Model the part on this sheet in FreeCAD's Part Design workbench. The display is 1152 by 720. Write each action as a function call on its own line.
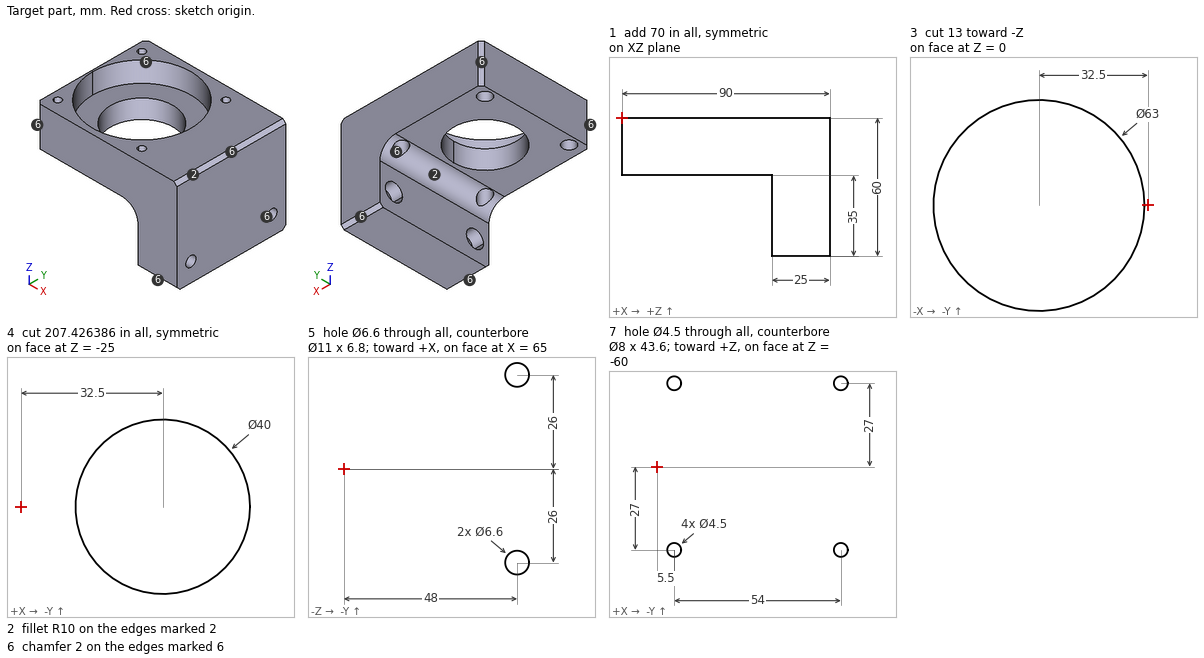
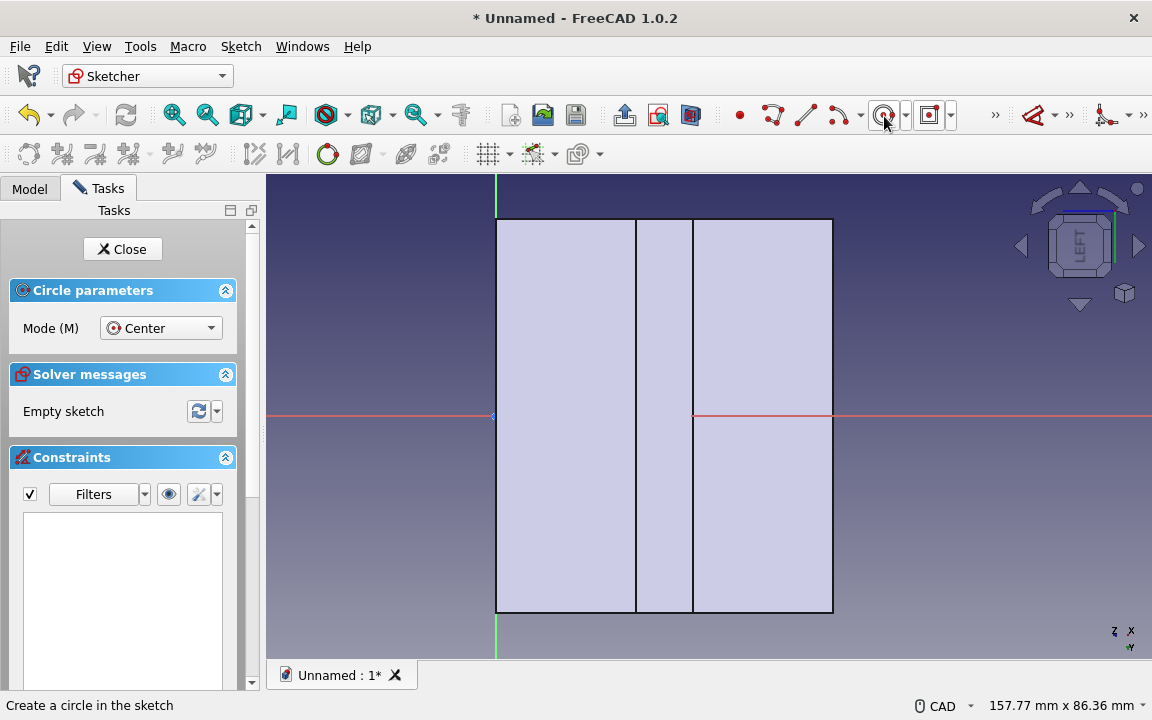
scroll(766, 562, up, 2)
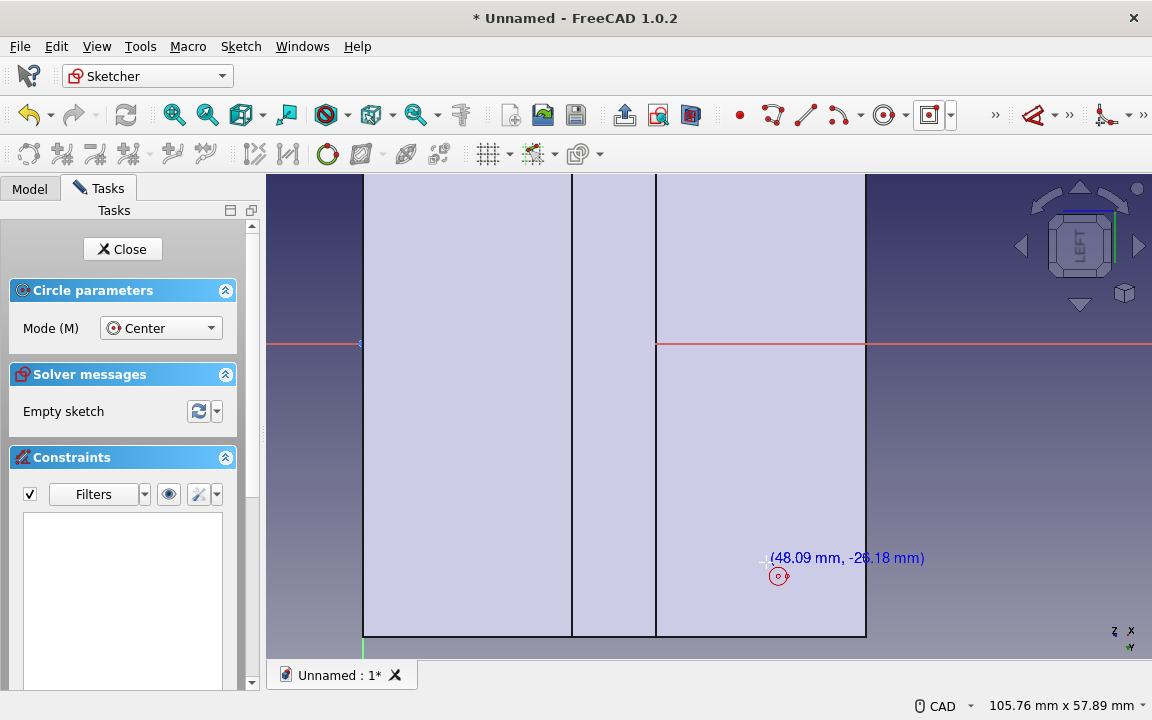
click(765, 562)
move(785, 542)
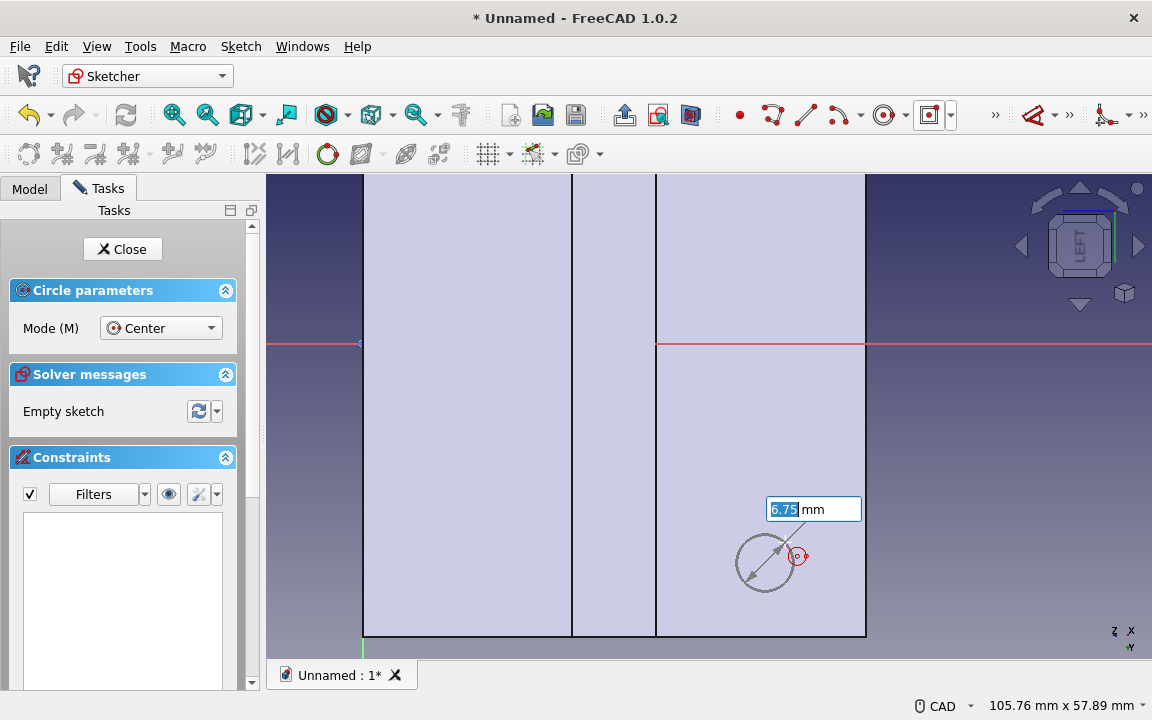
text(6.6)
key(Return)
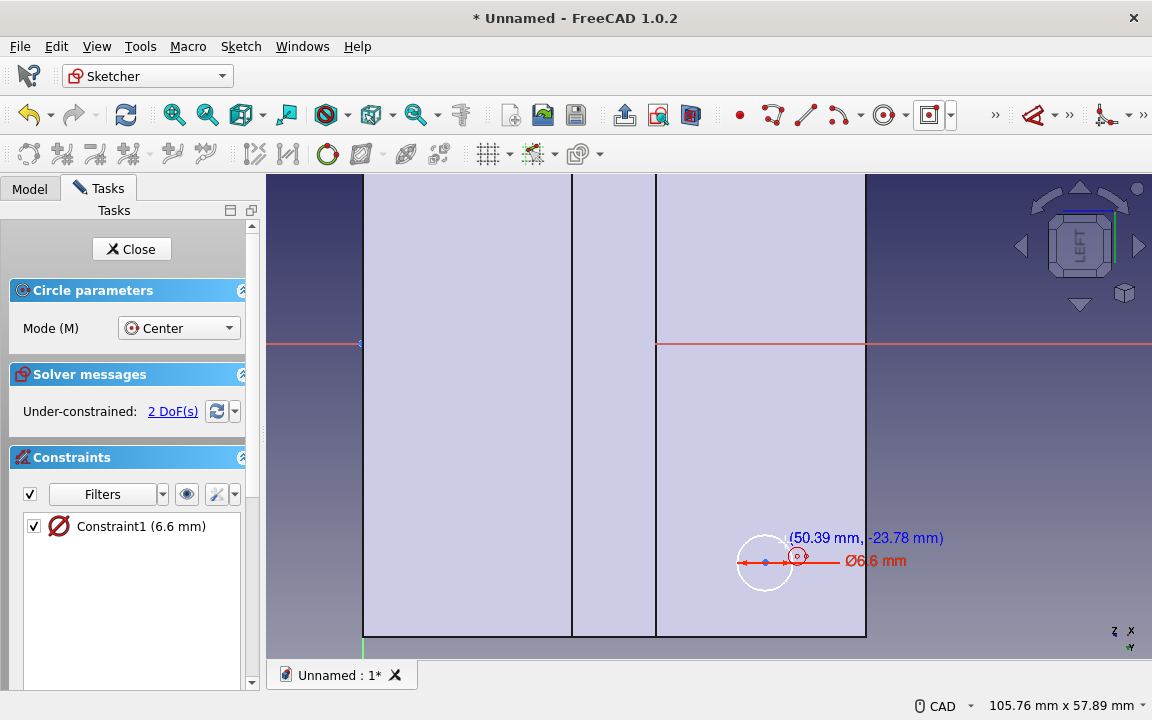
scroll(768, 564, down, 2)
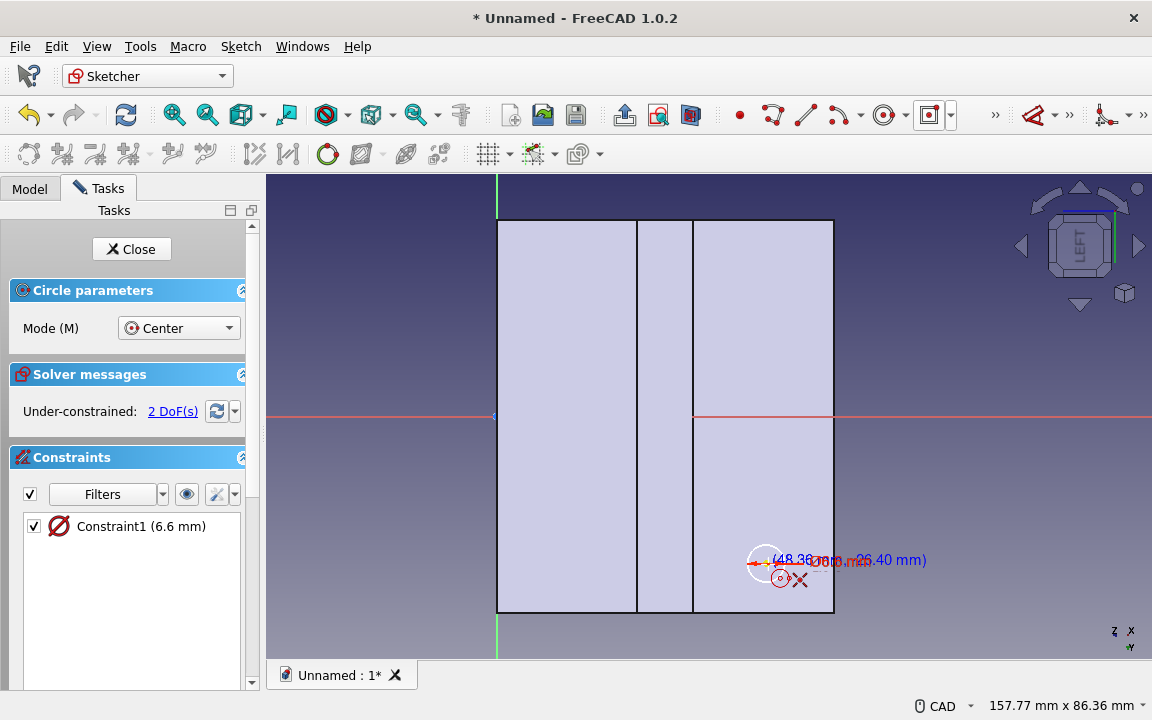
scroll(766, 271, up, 2)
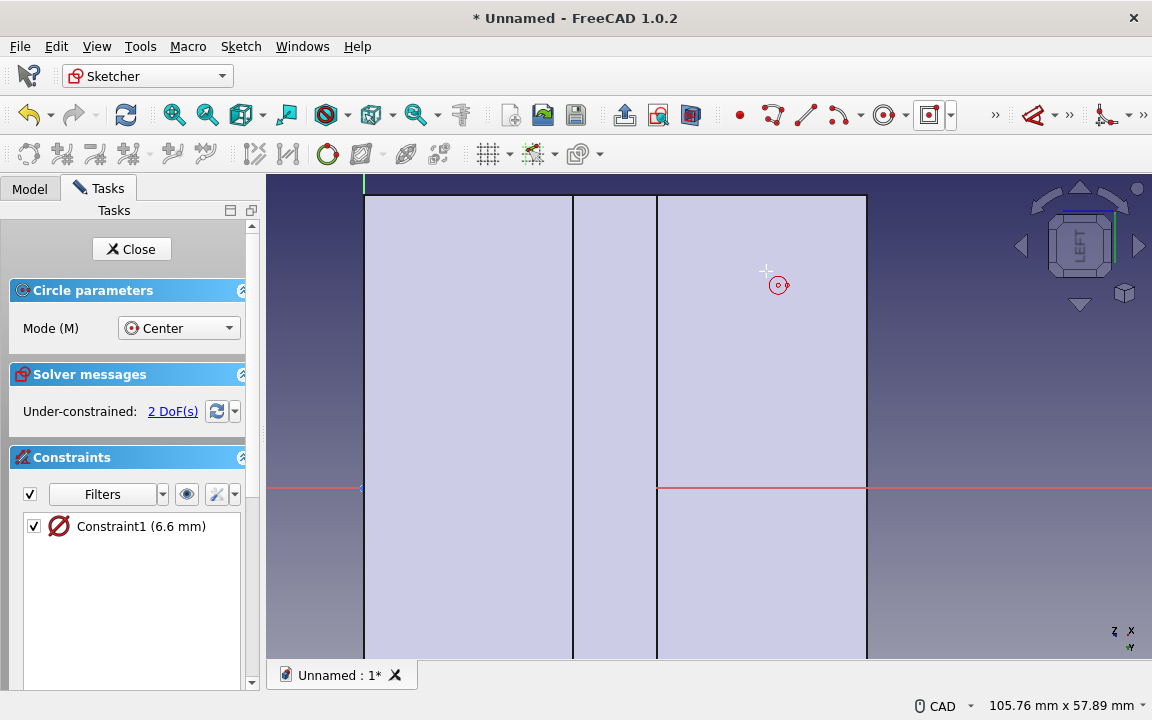
click(766, 270)
move(786, 251)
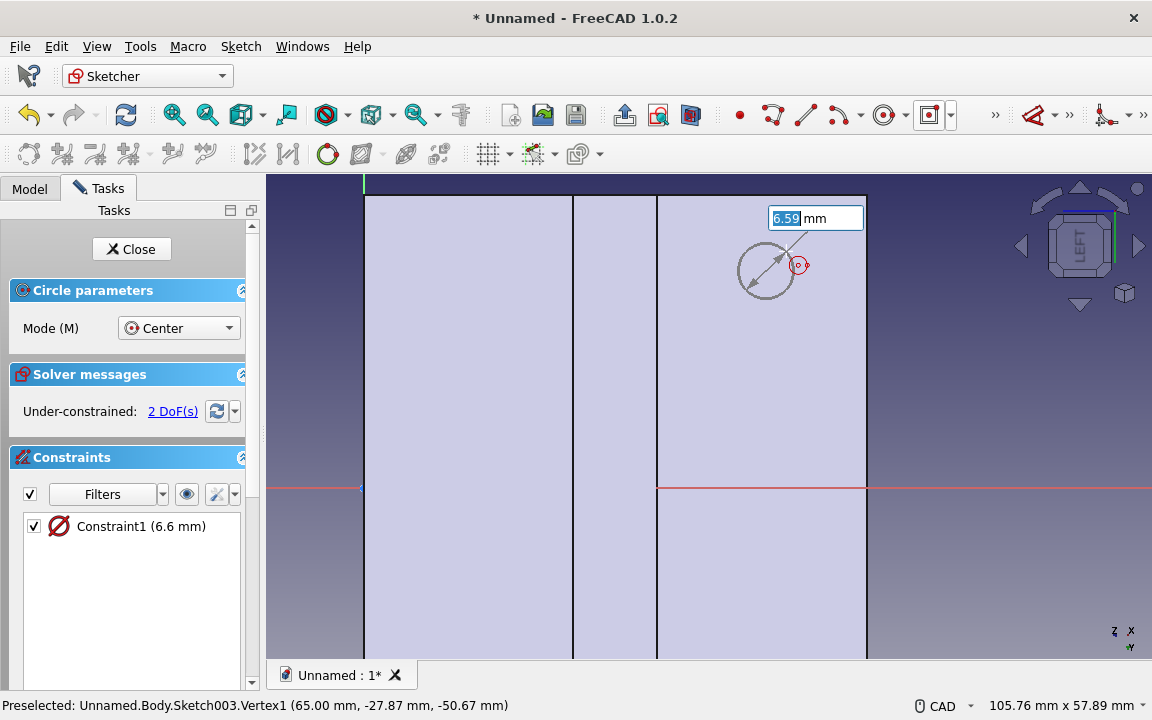
text(6.6)
key(Return)
key(Escape)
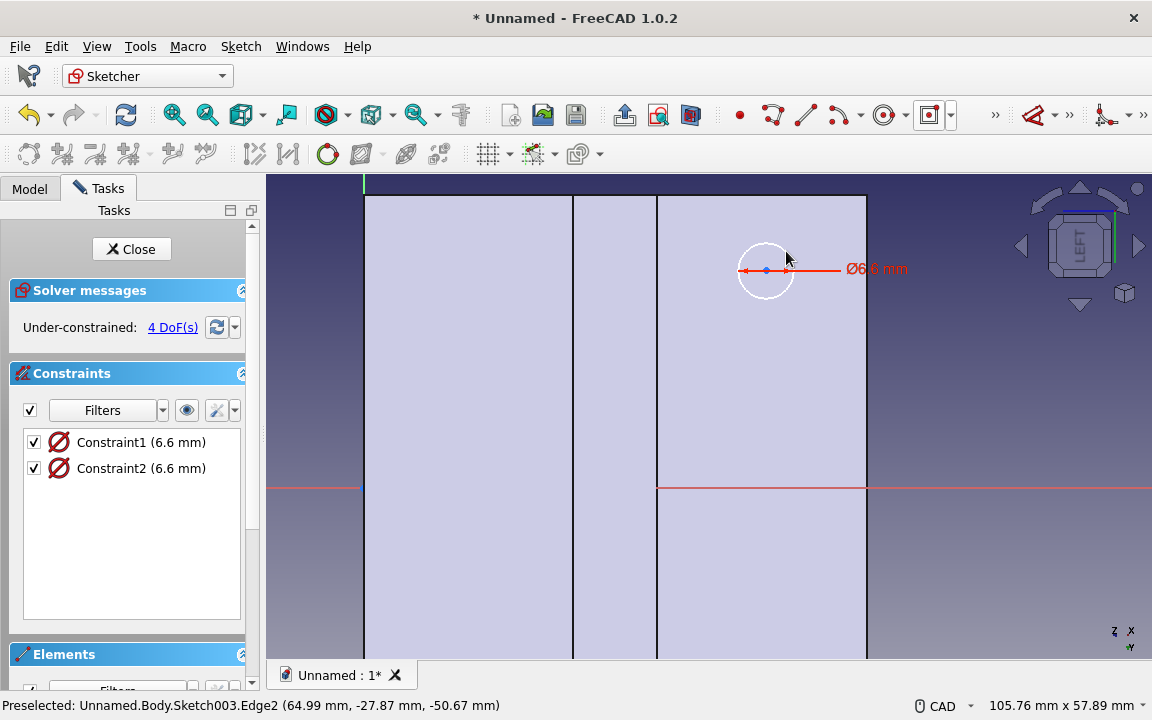
scroll(766, 271, down, 2)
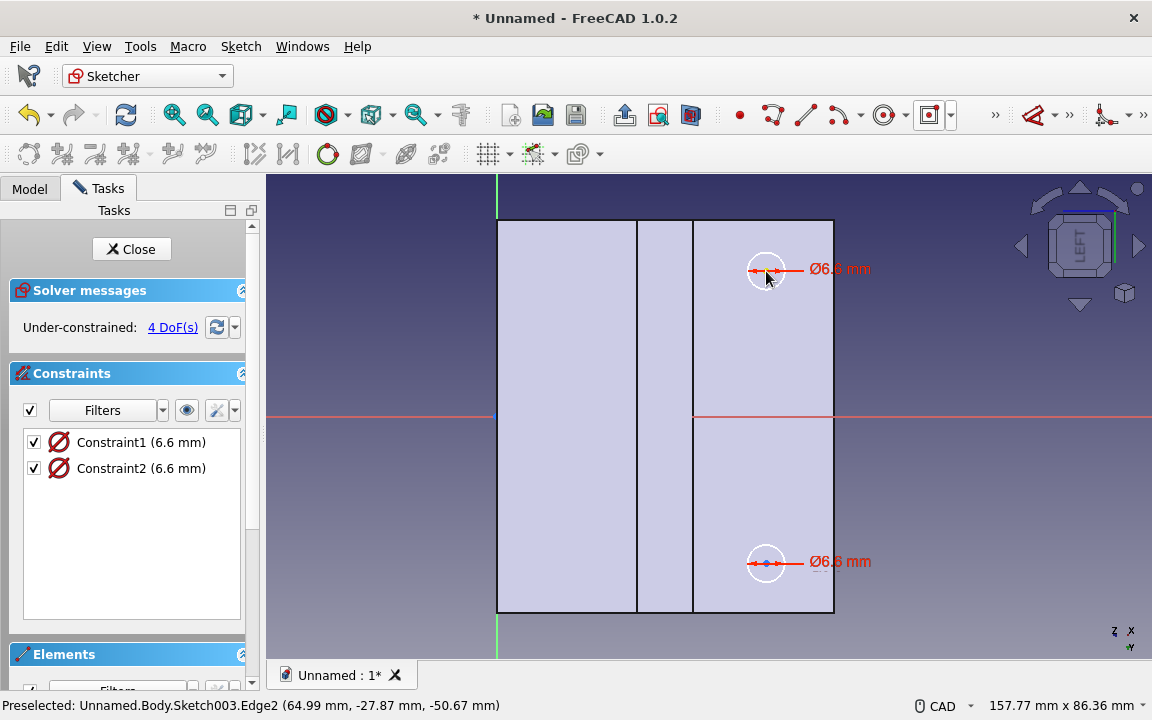
click(766, 564)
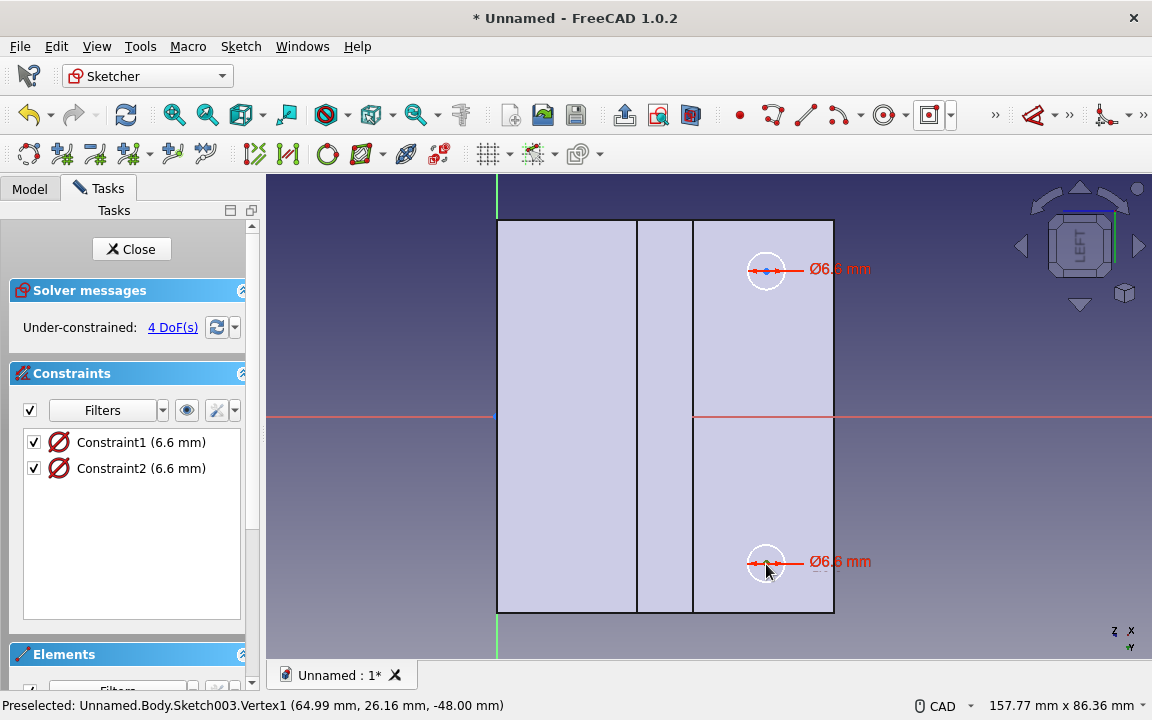
click(766, 271)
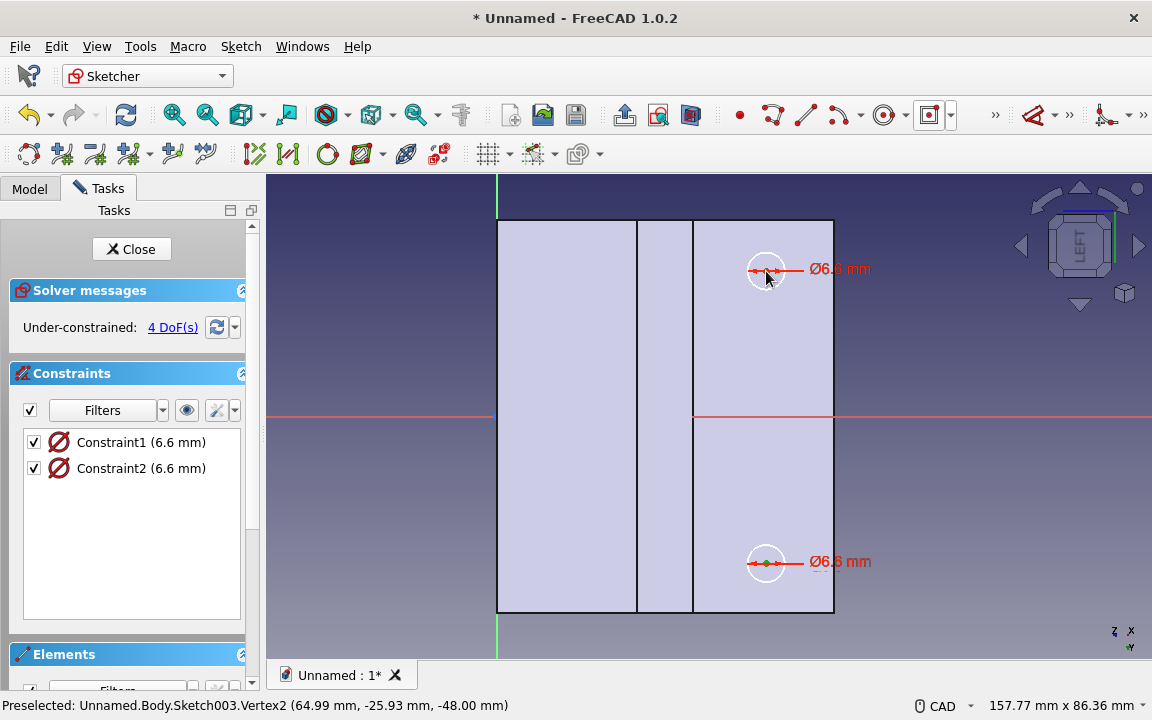
key(v)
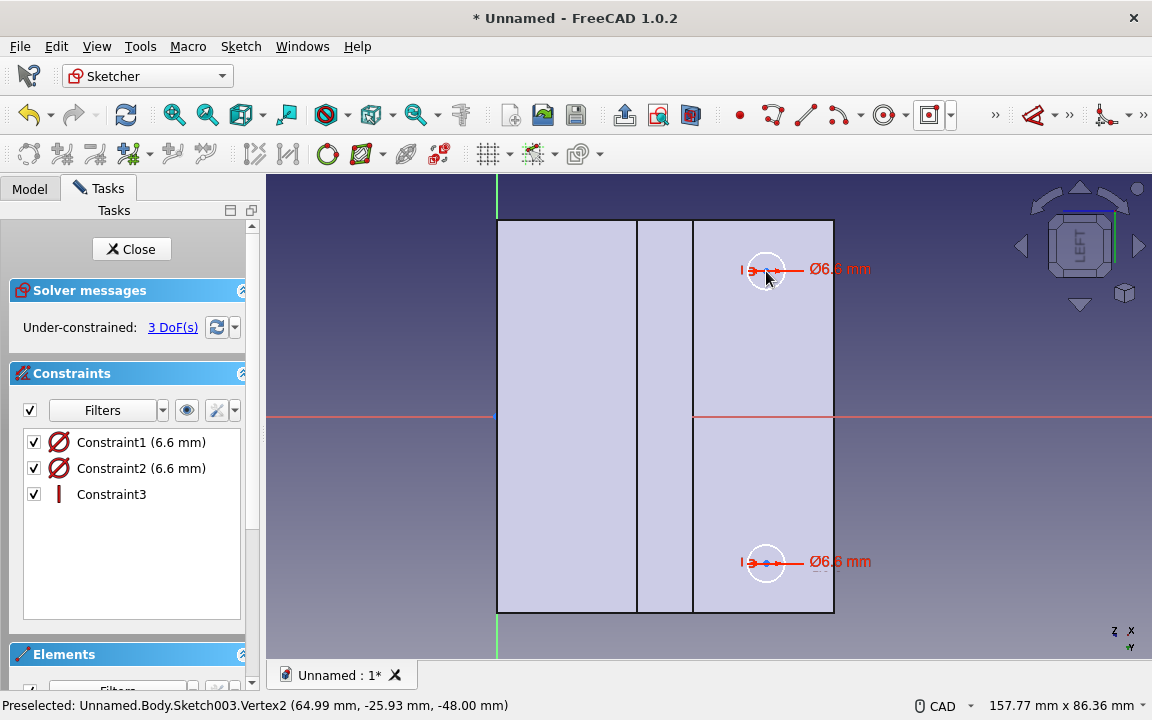
click(1032, 116)